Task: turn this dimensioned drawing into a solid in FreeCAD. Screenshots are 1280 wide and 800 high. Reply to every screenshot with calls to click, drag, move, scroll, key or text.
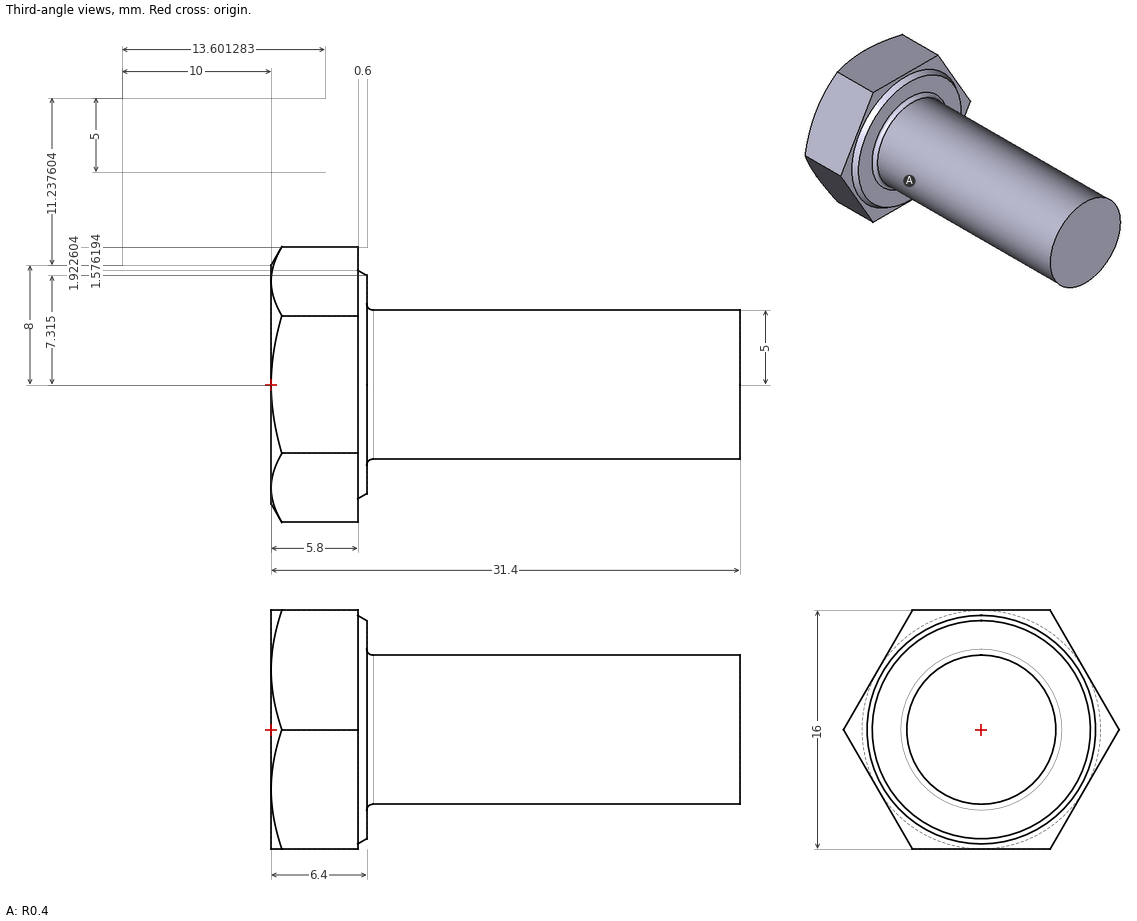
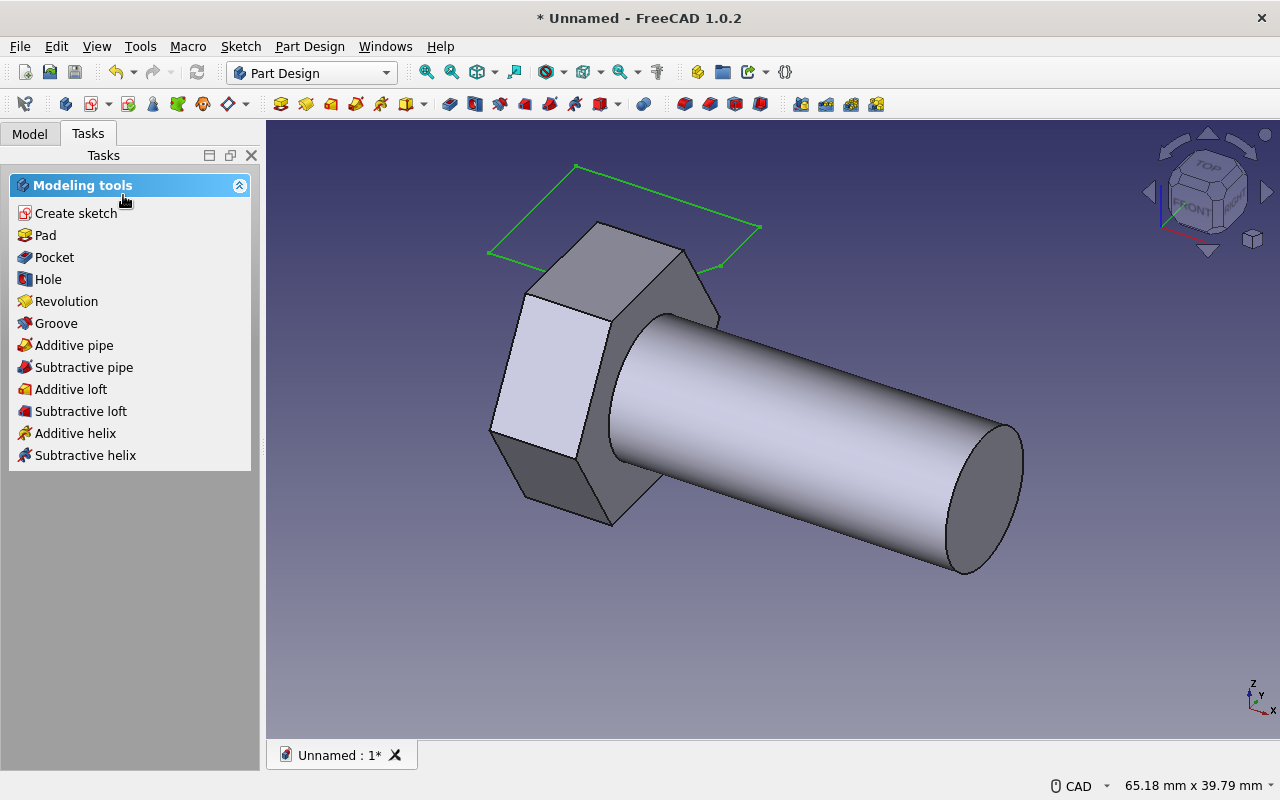
click(500, 104)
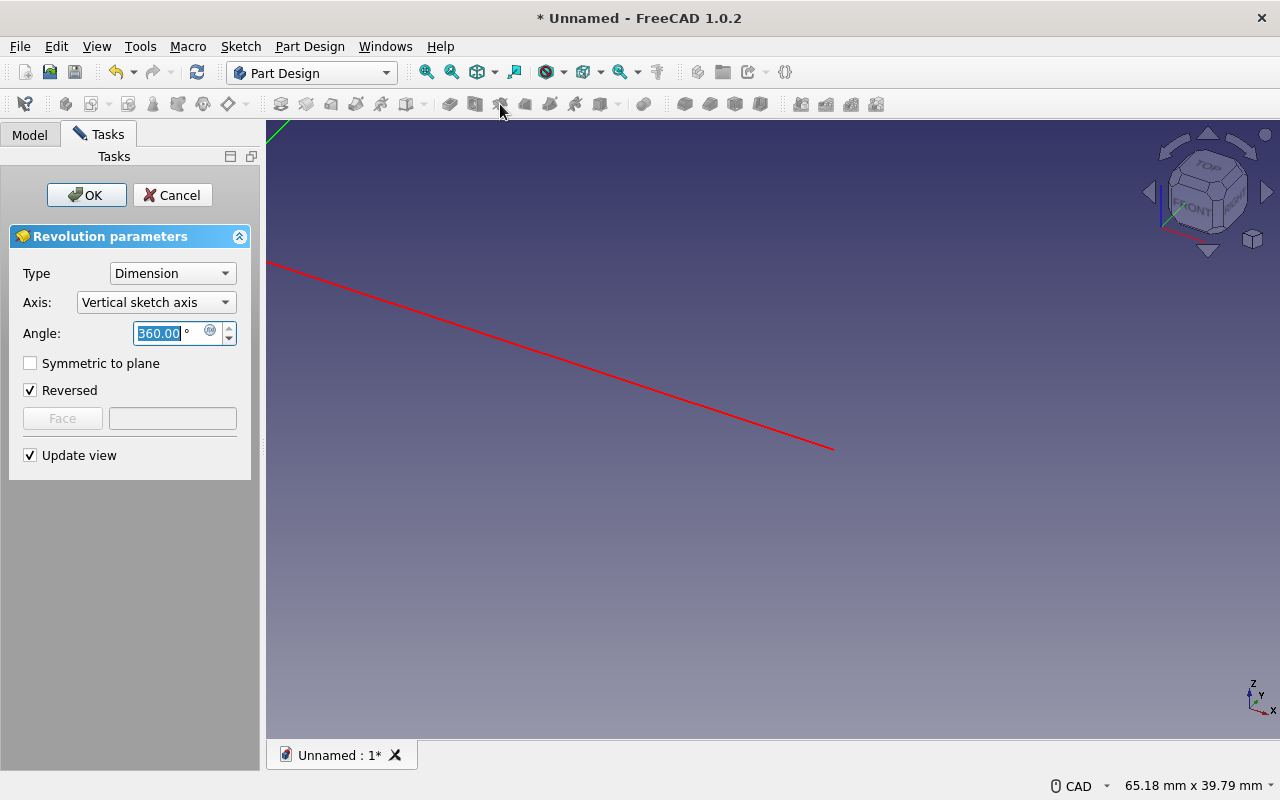
click(157, 302)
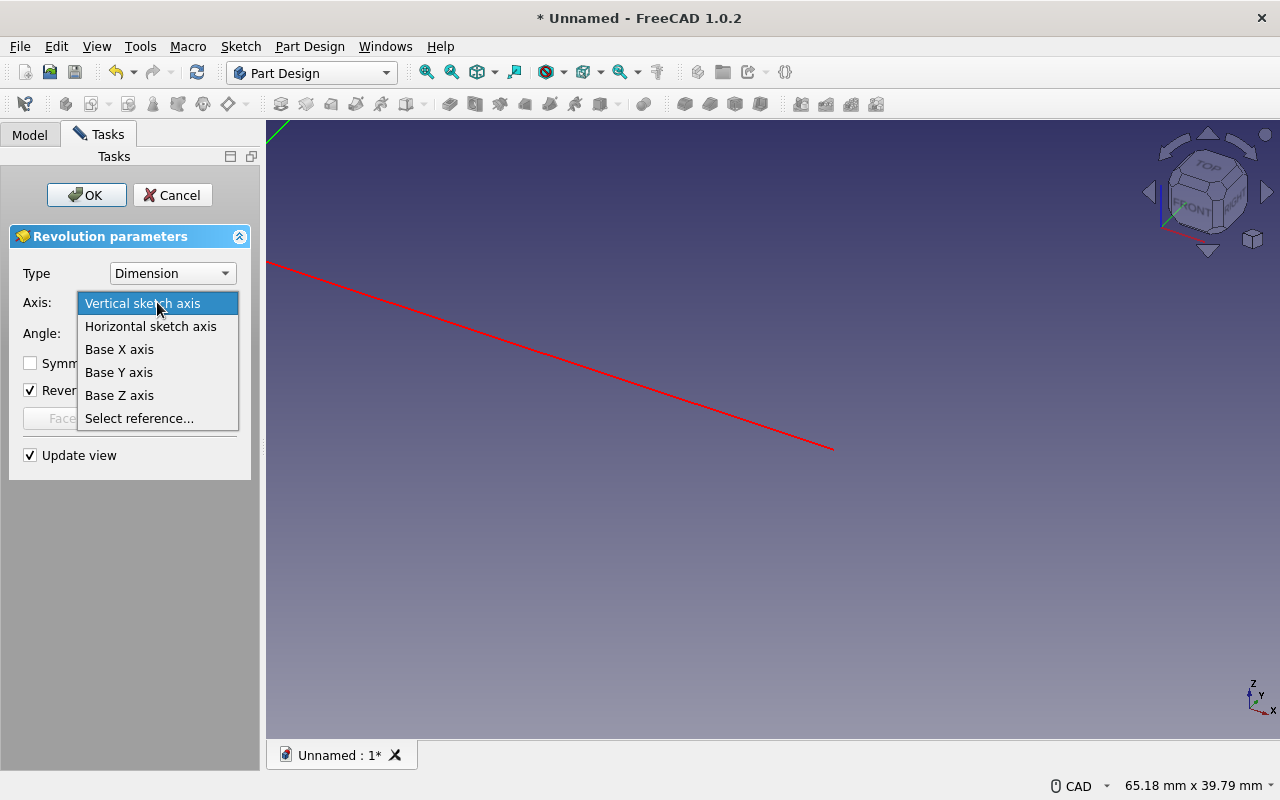
click(156, 326)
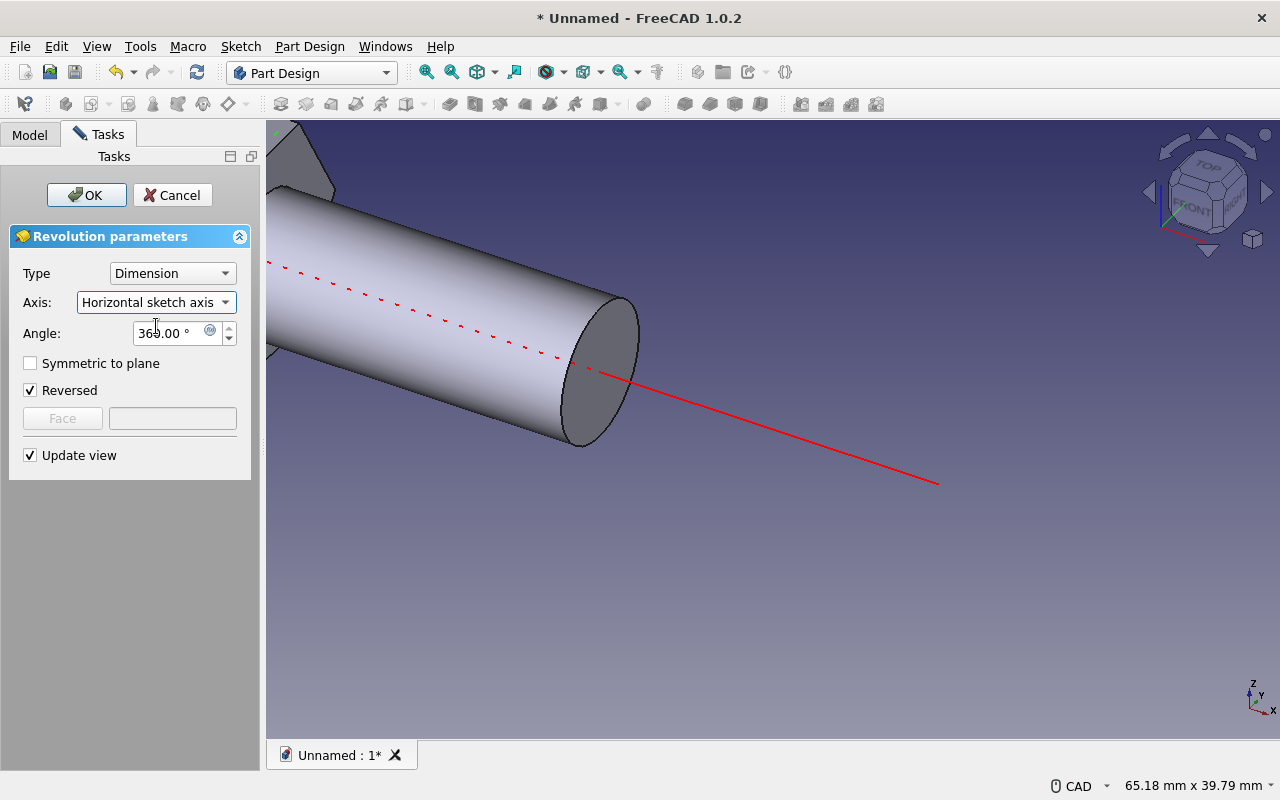
click(87, 195)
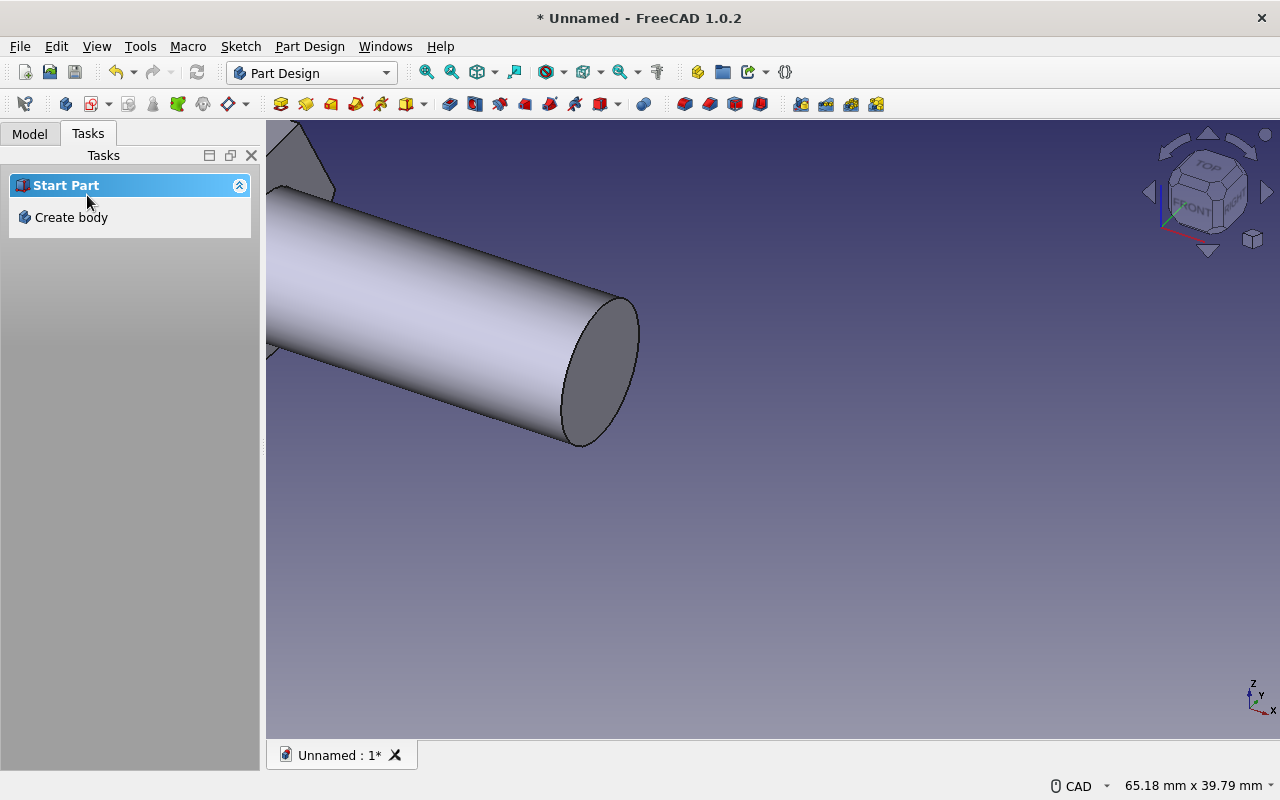
click(427, 72)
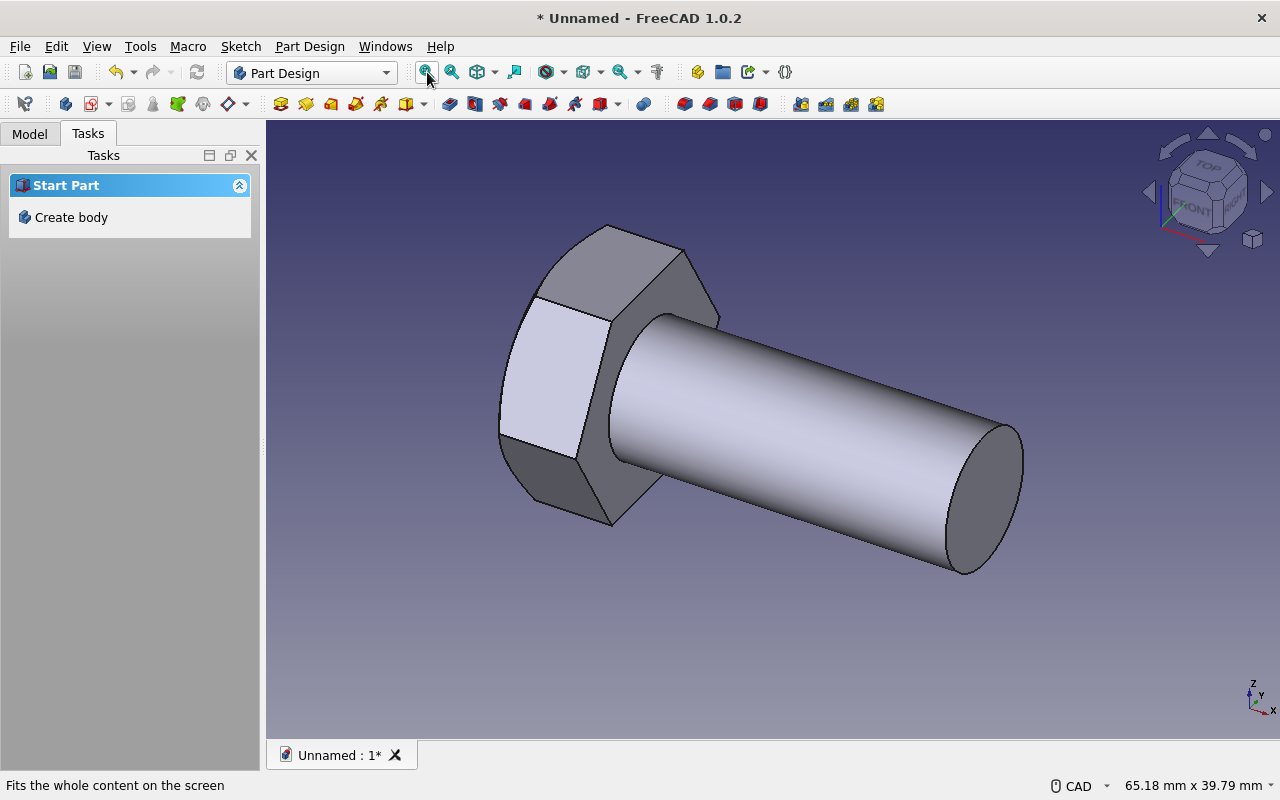
click(90, 104)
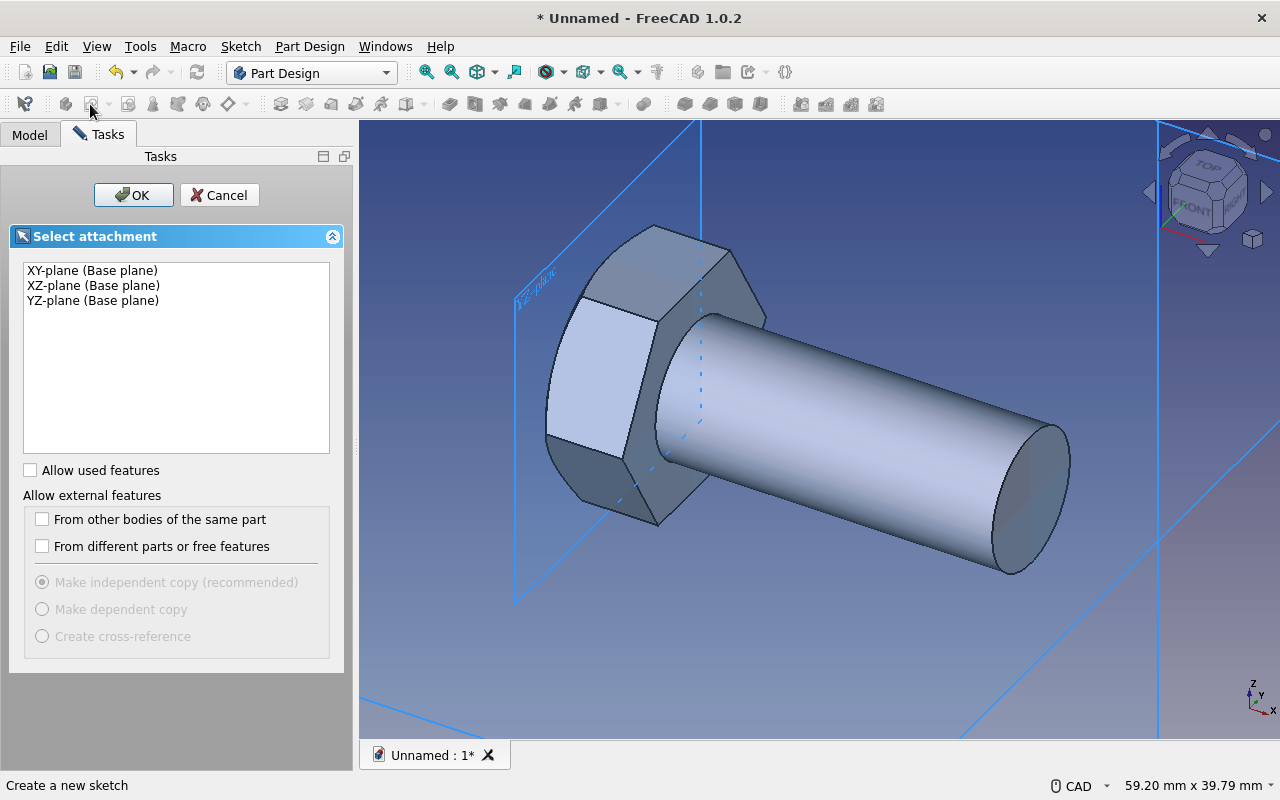
click(84, 270)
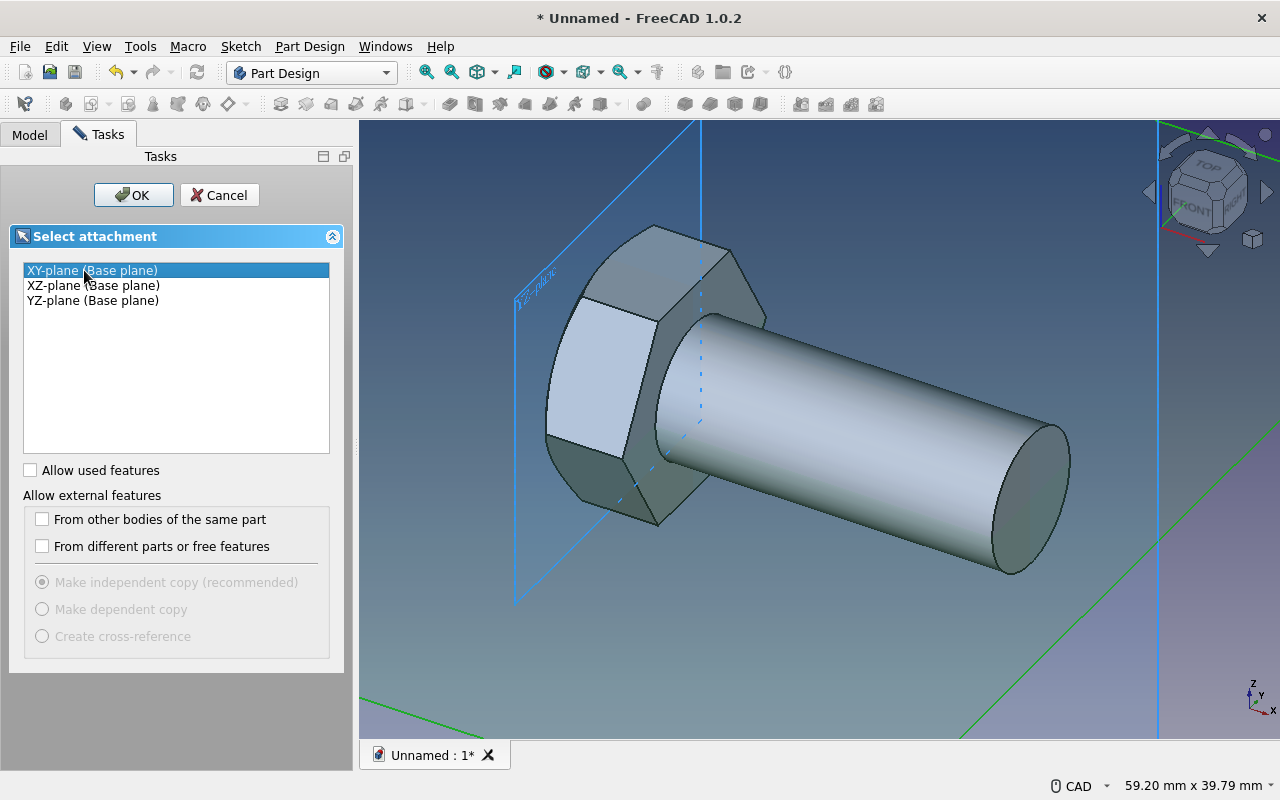
click(134, 195)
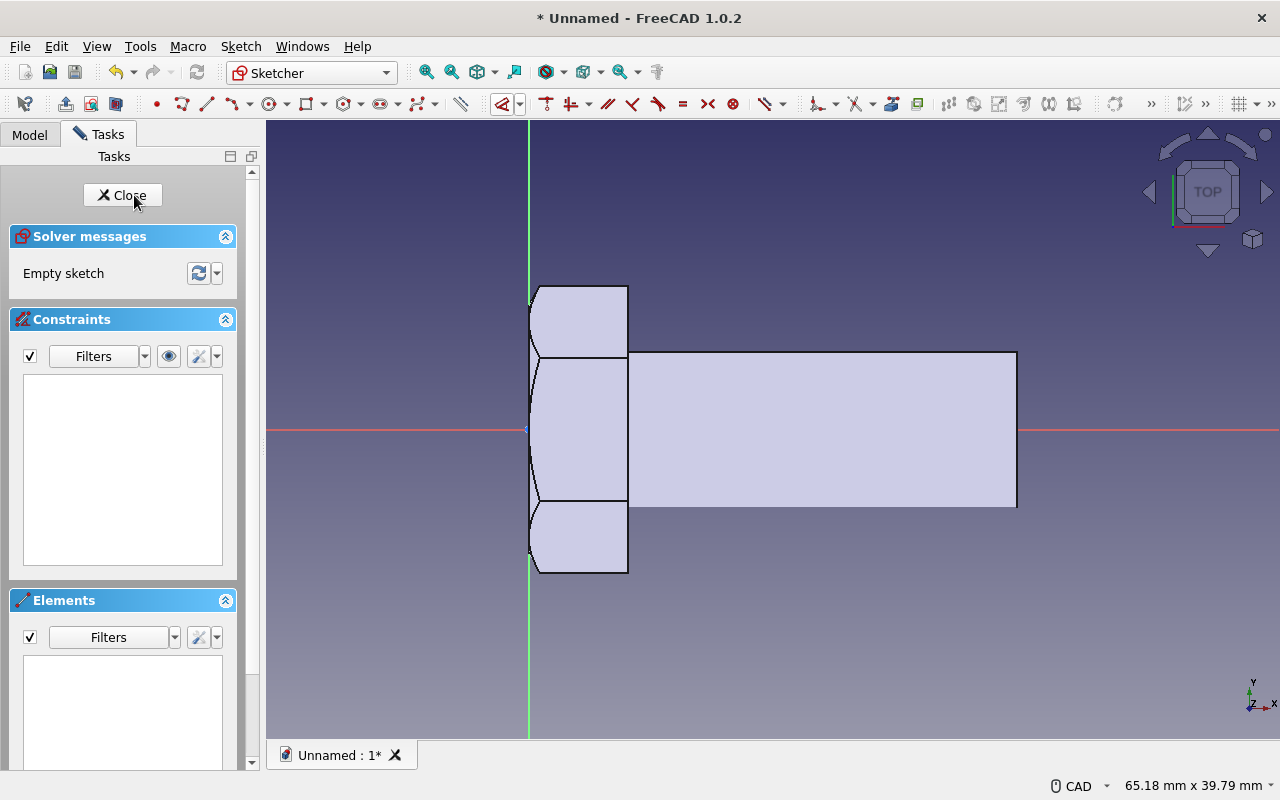
key(q)
key(s)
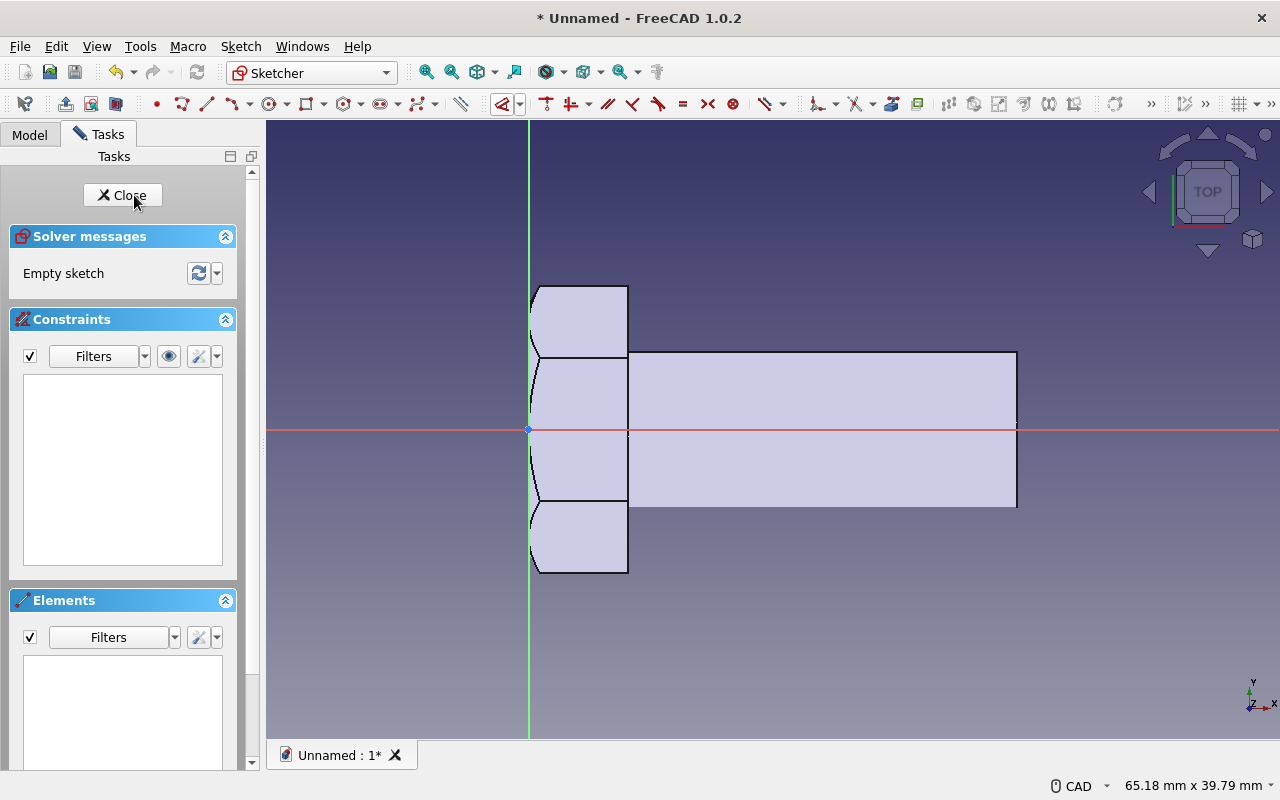
scroll(617, 290, up, 13)